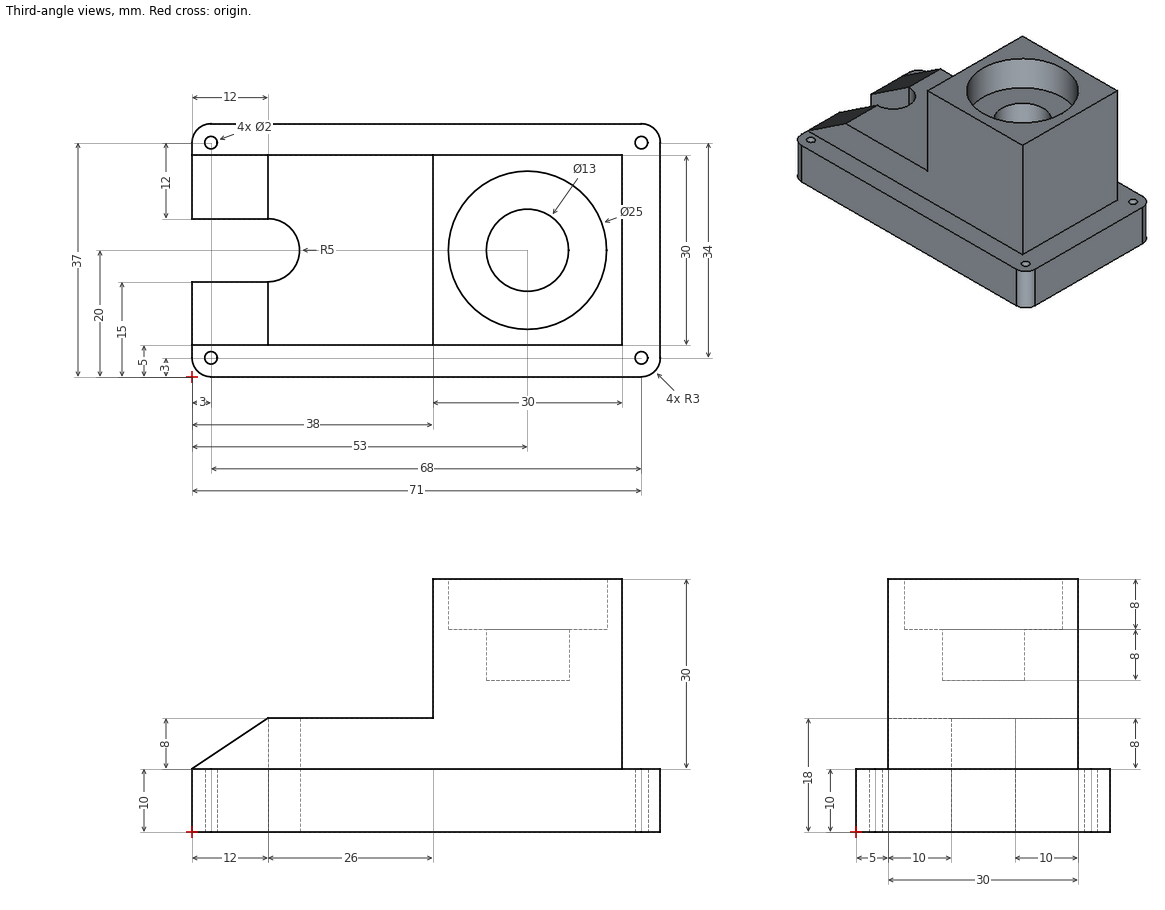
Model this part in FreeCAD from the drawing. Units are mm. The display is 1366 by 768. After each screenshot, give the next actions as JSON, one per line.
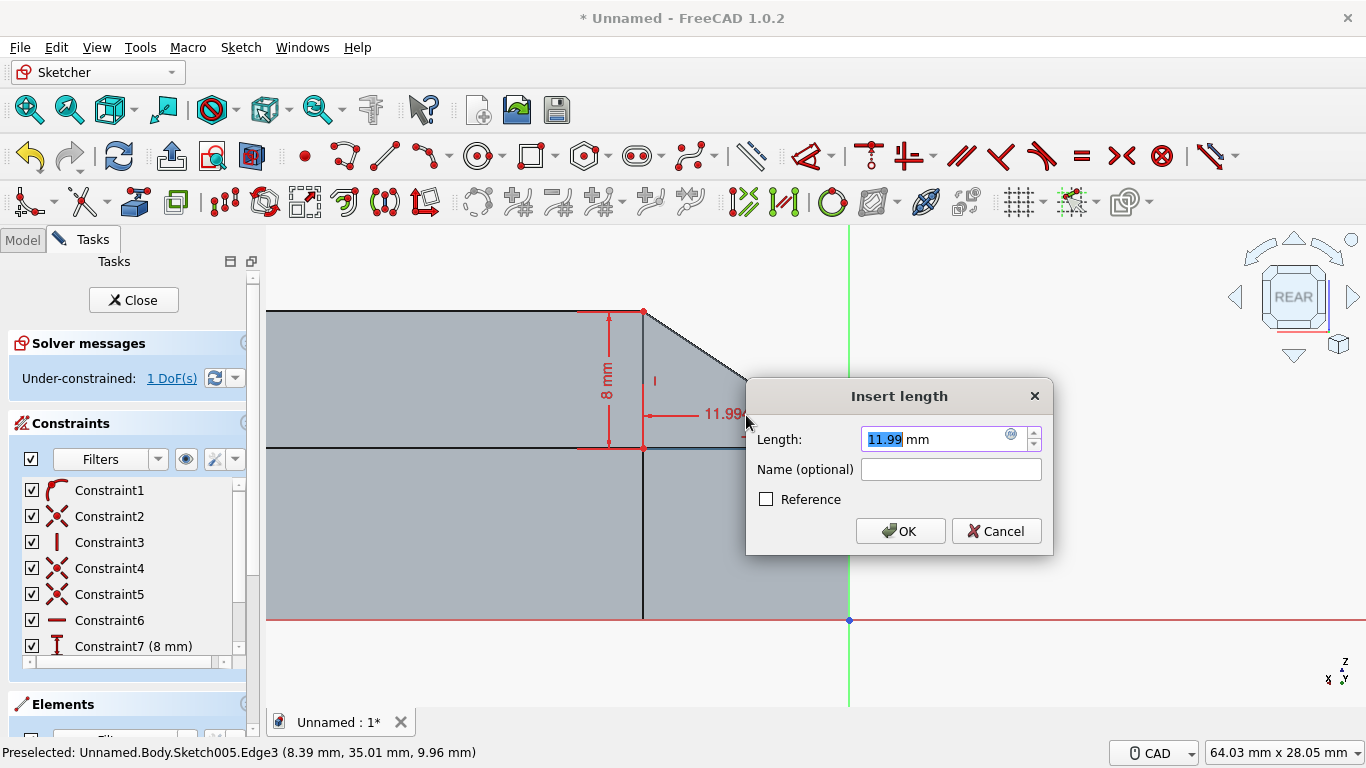
{"action": "type", "text": "12"}
{"action": "key", "text": "Return"}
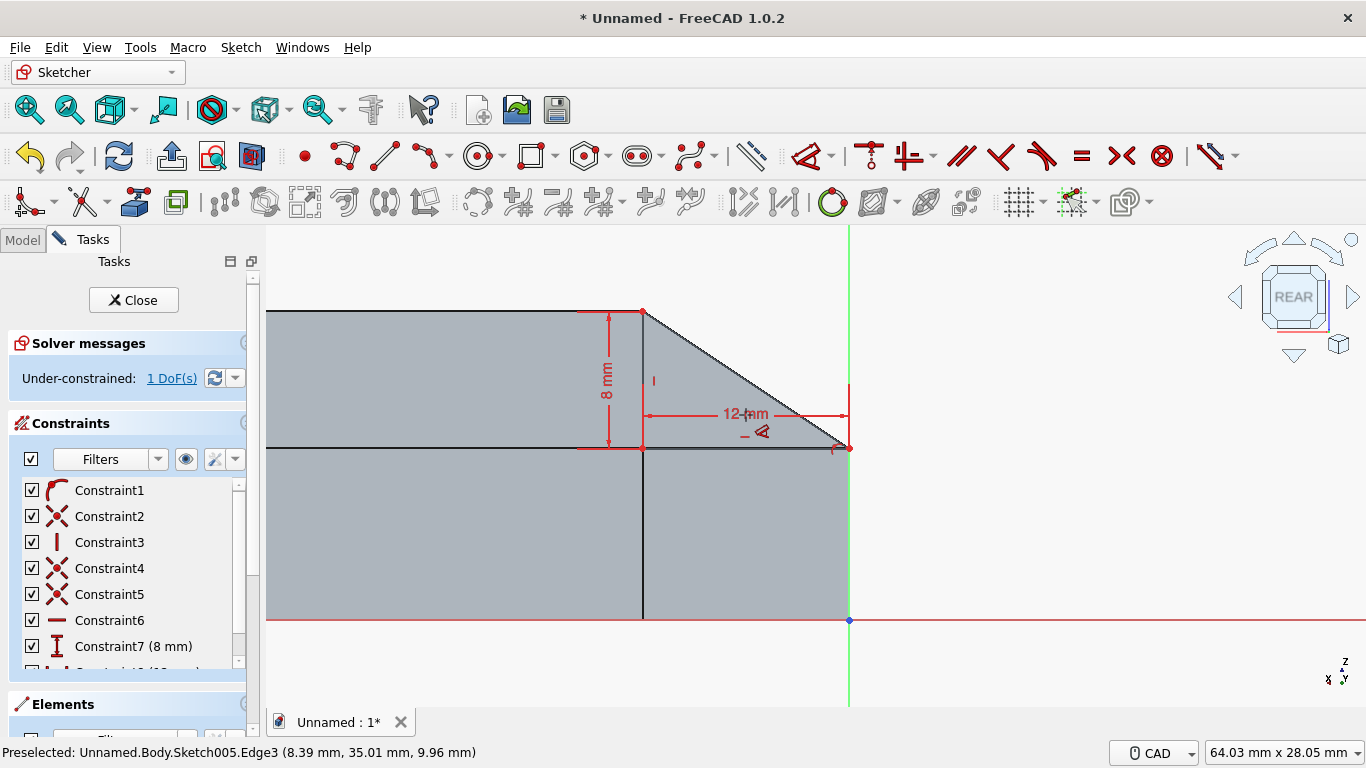
{"action": "left_click", "coordinate": [849, 449]}
{"action": "left_click", "coordinate": [883, 535]}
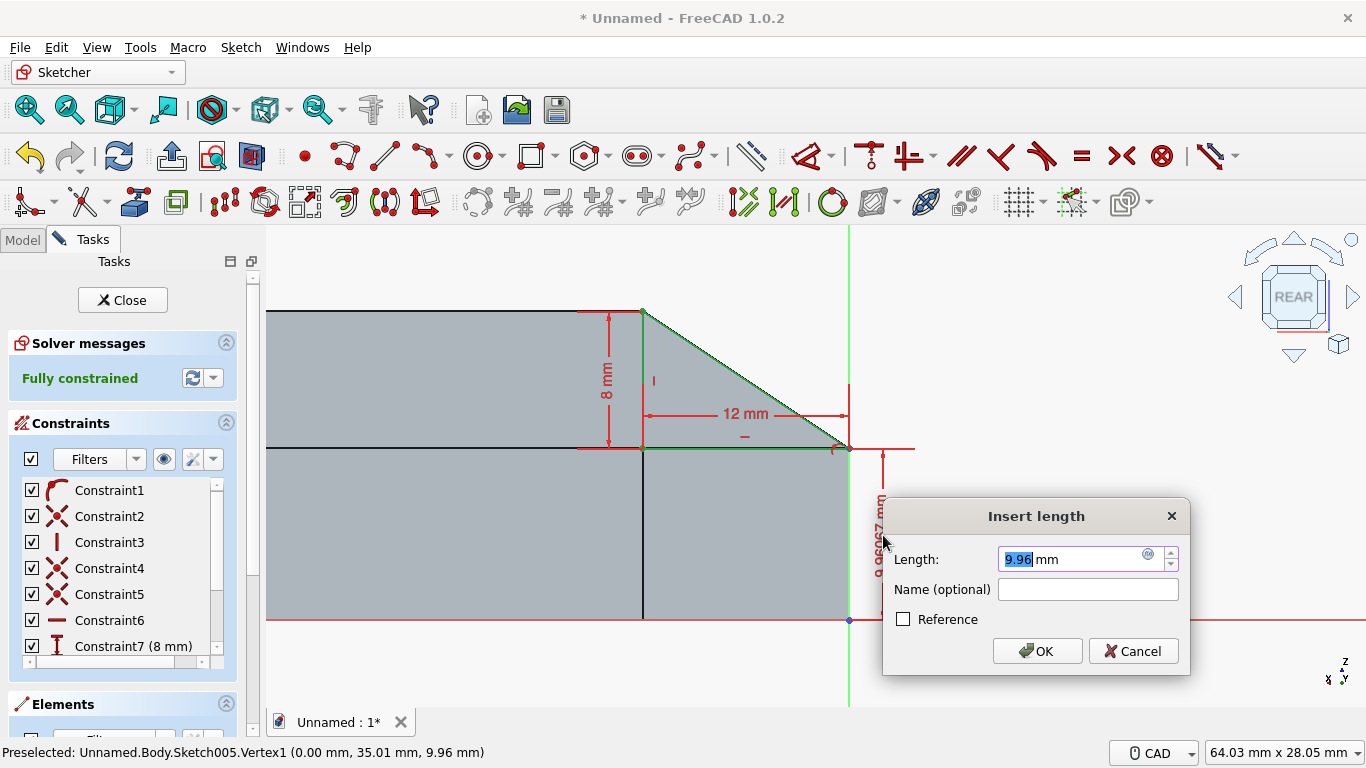
{"action": "type", "text": "10"}
{"action": "key", "text": "Return"}
{"action": "key", "text": "Escape"}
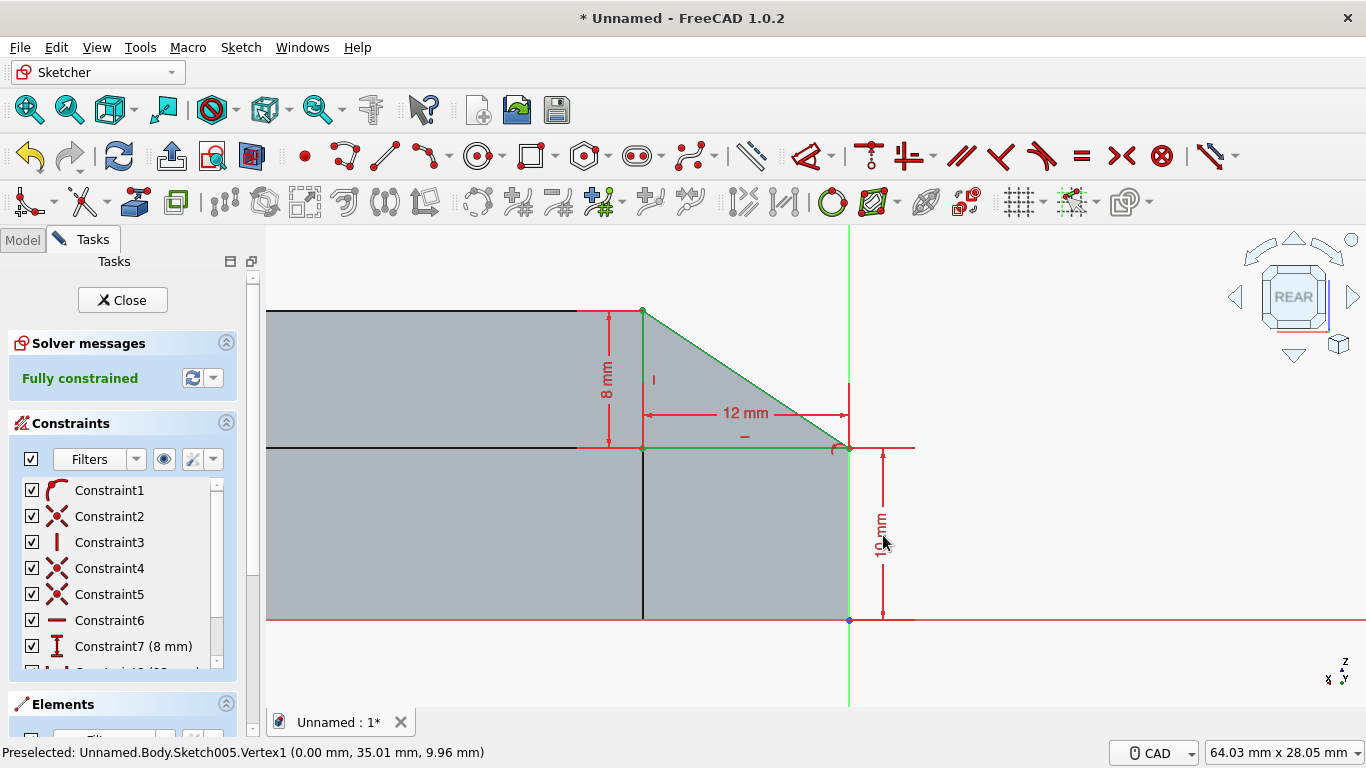
{"action": "left_click", "coordinate": [123, 300]}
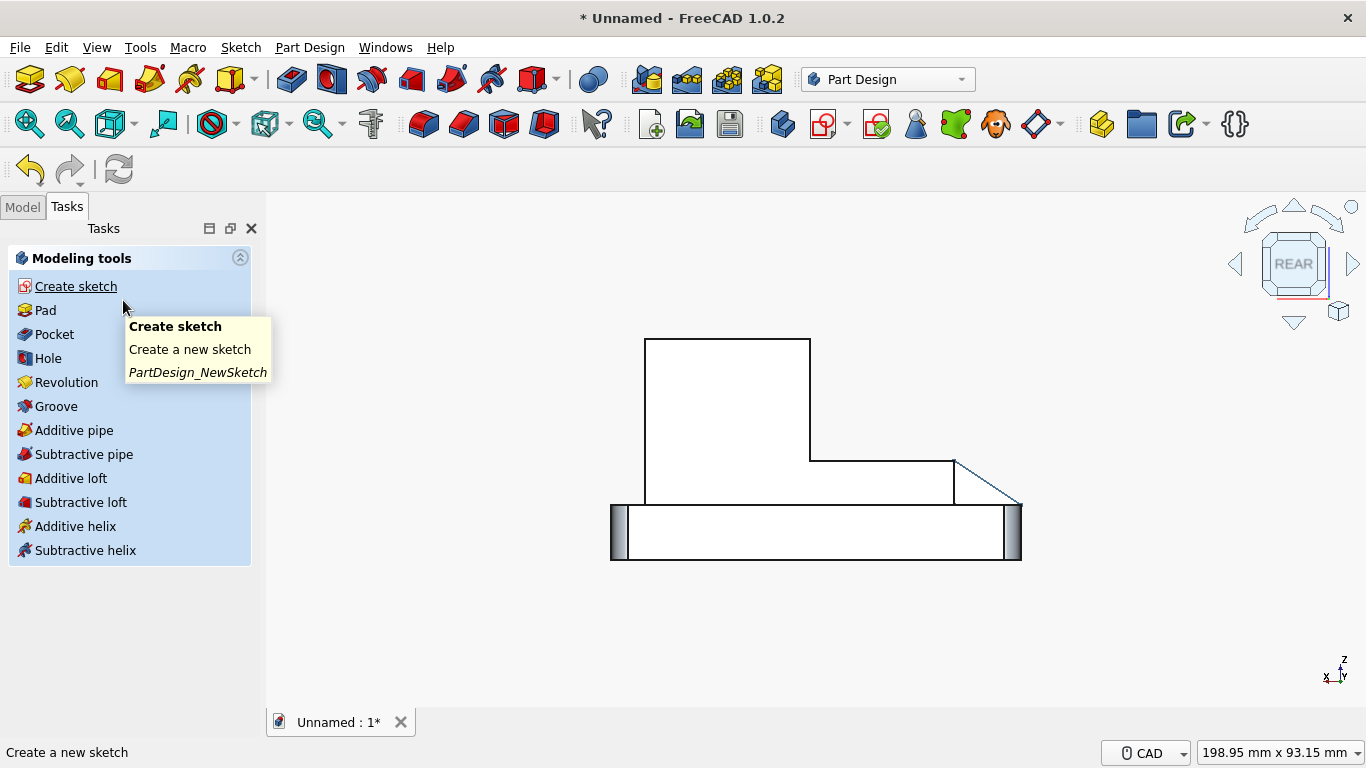
{"action": "left_click", "coordinate": [30, 80]}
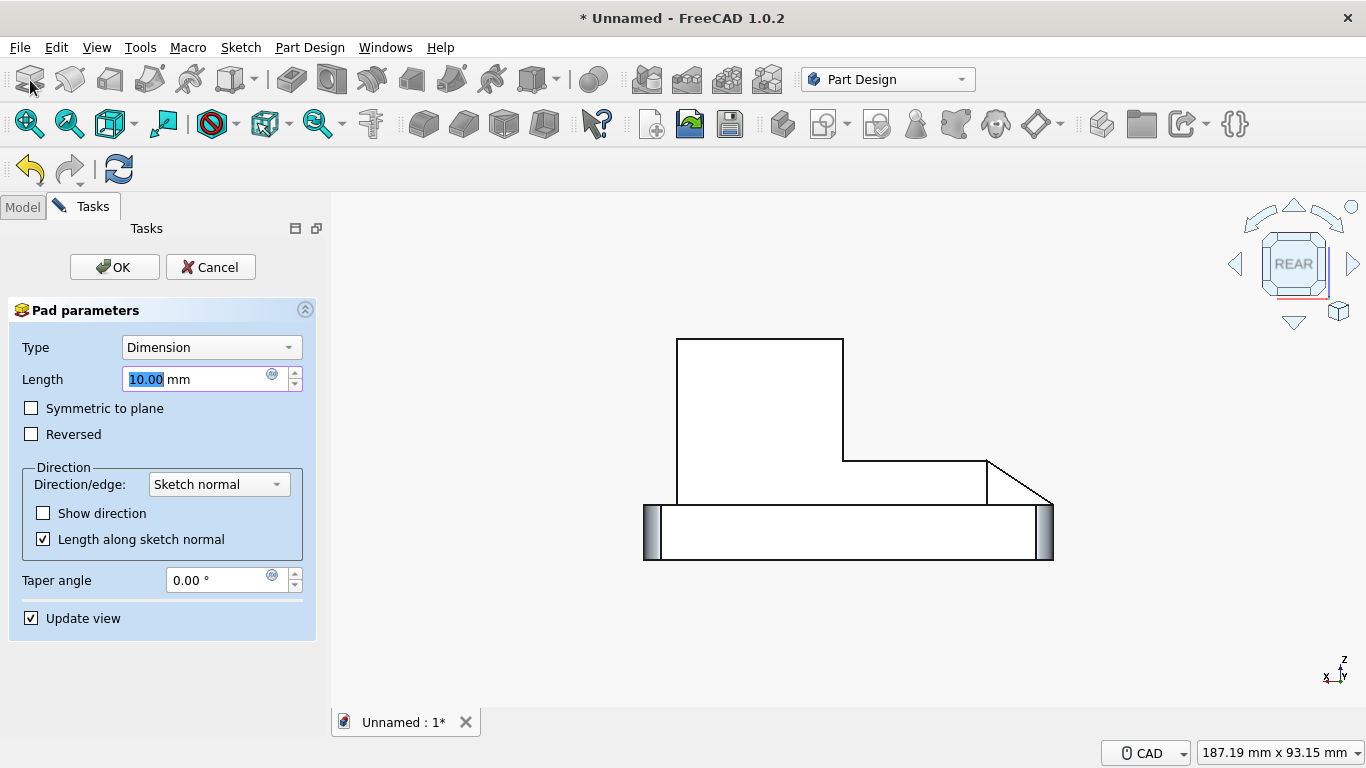
{"action": "type", "text": "10"}
{"action": "key", "text": "Tab"}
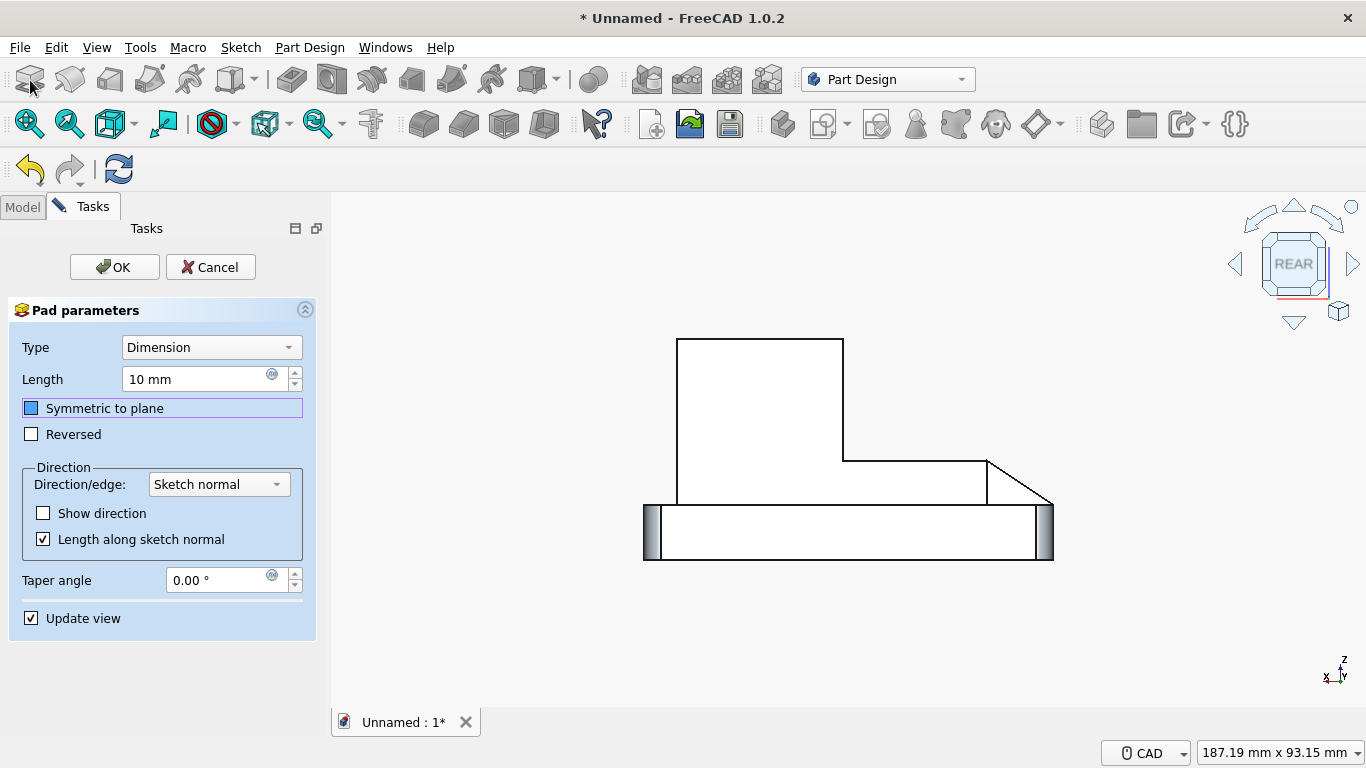
{"action": "left_click", "coordinate": [30, 434]}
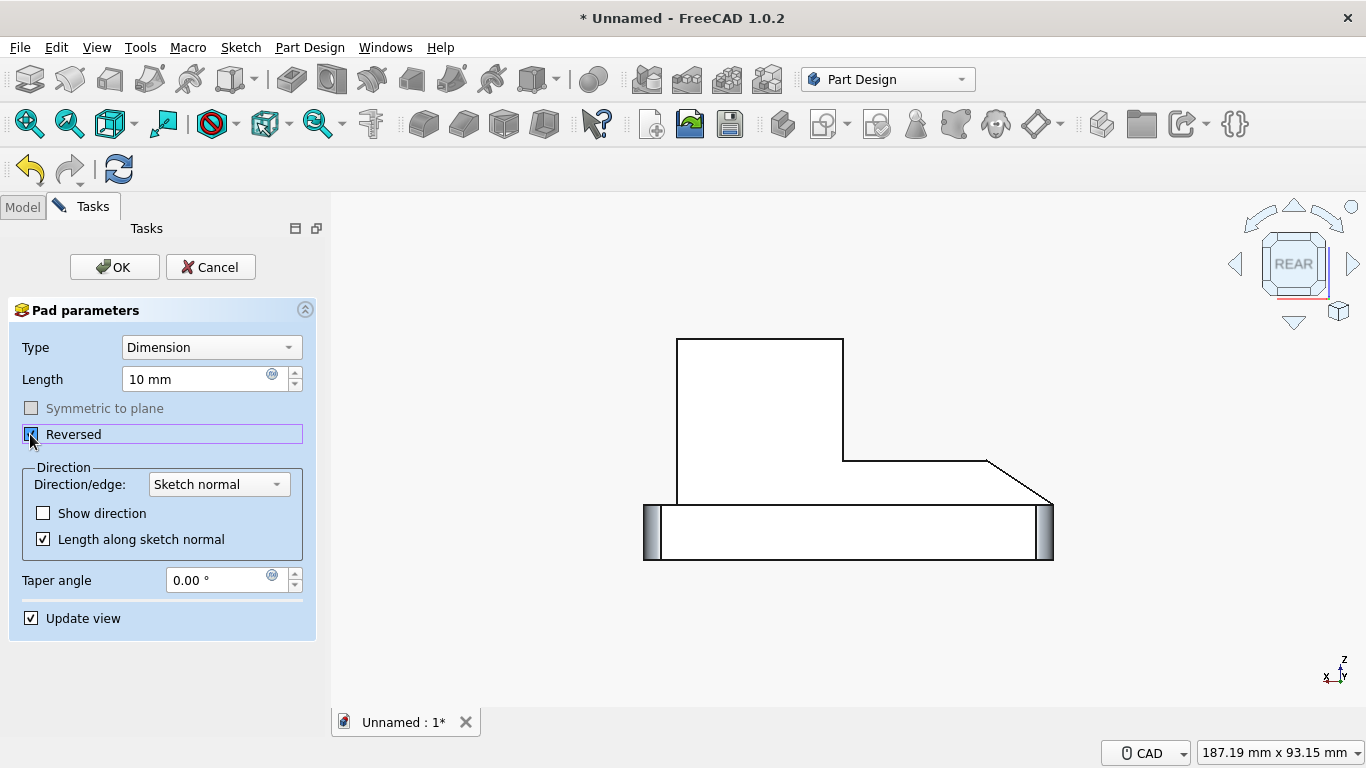
{"action": "left_click", "coordinate": [115, 267]}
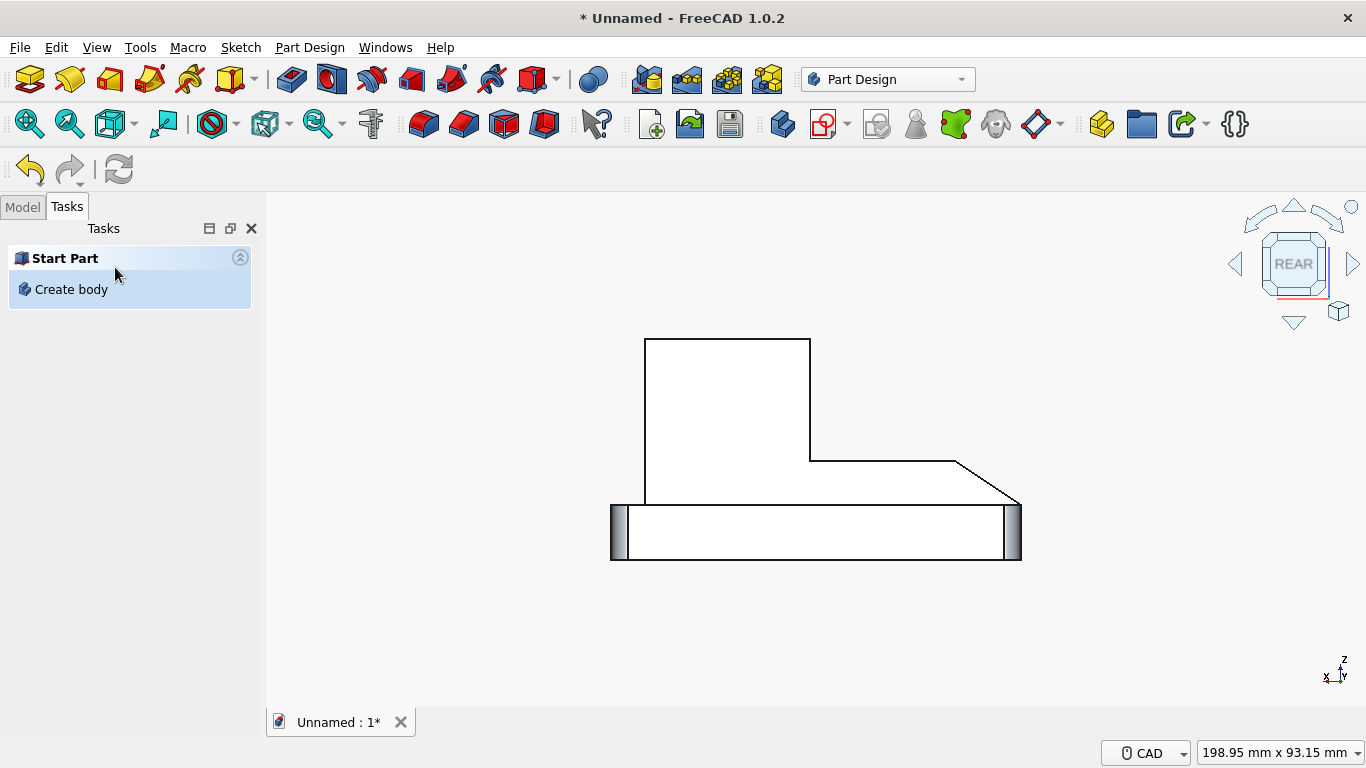
{"action": "left_click", "coordinate": [30, 124]}